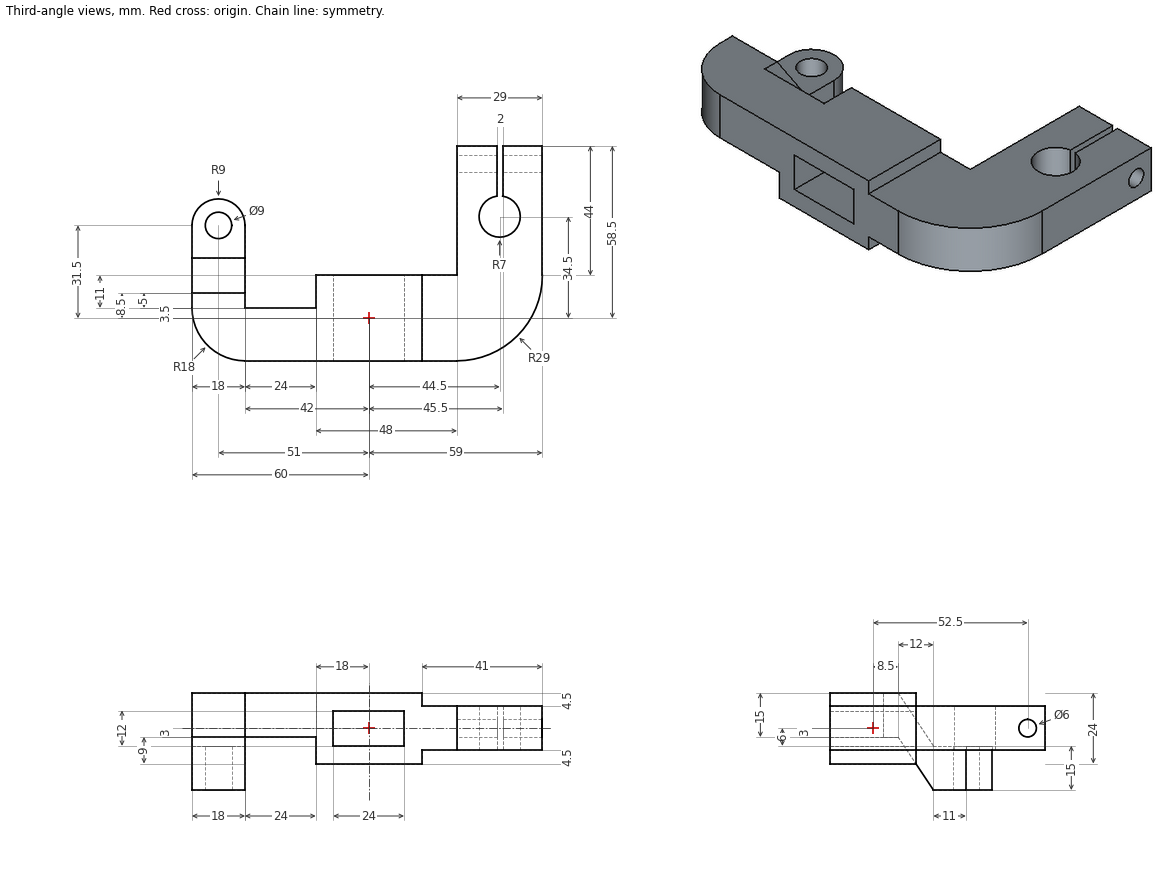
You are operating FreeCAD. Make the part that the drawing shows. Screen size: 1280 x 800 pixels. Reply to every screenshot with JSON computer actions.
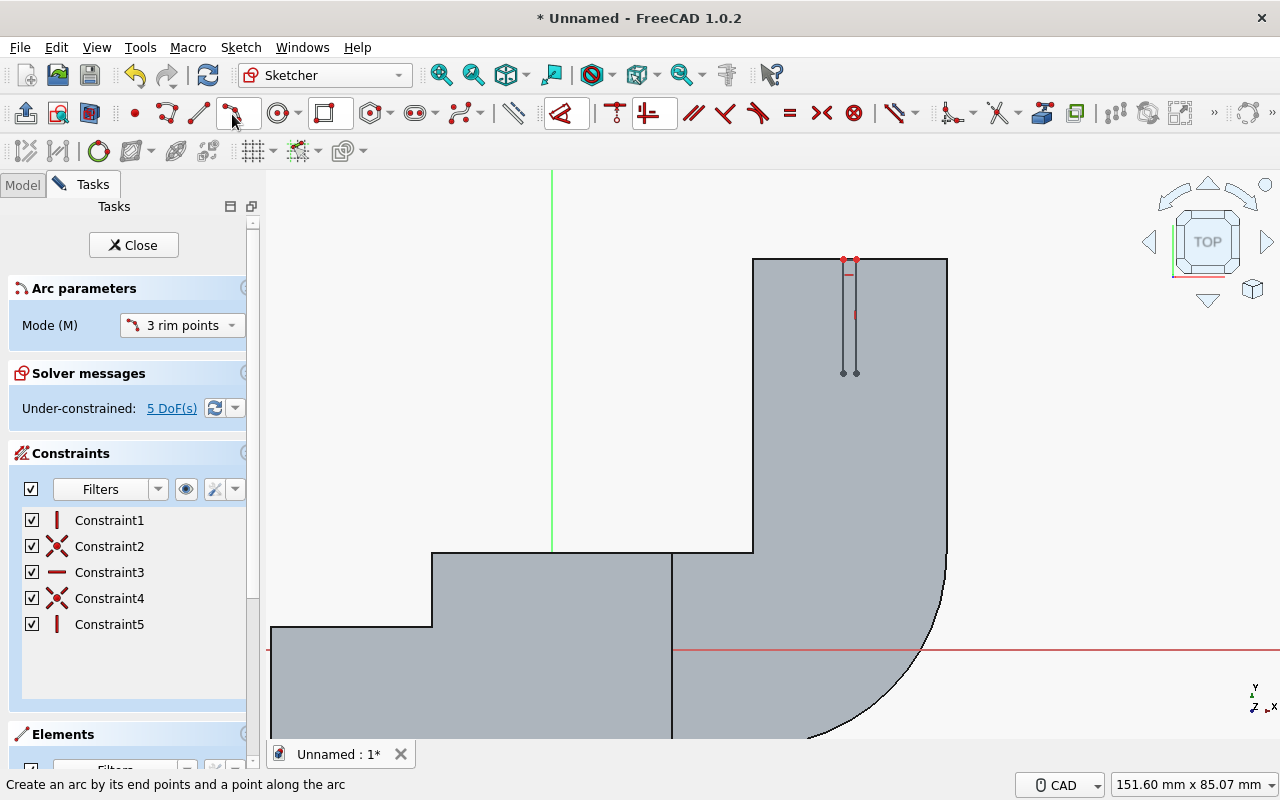
{"action": "left_click", "coordinate": [843, 374]}
{"action": "left_click", "coordinate": [856, 374]}
{"action": "left_click", "coordinate": [850, 466]}
{"action": "key", "text": "Escape"}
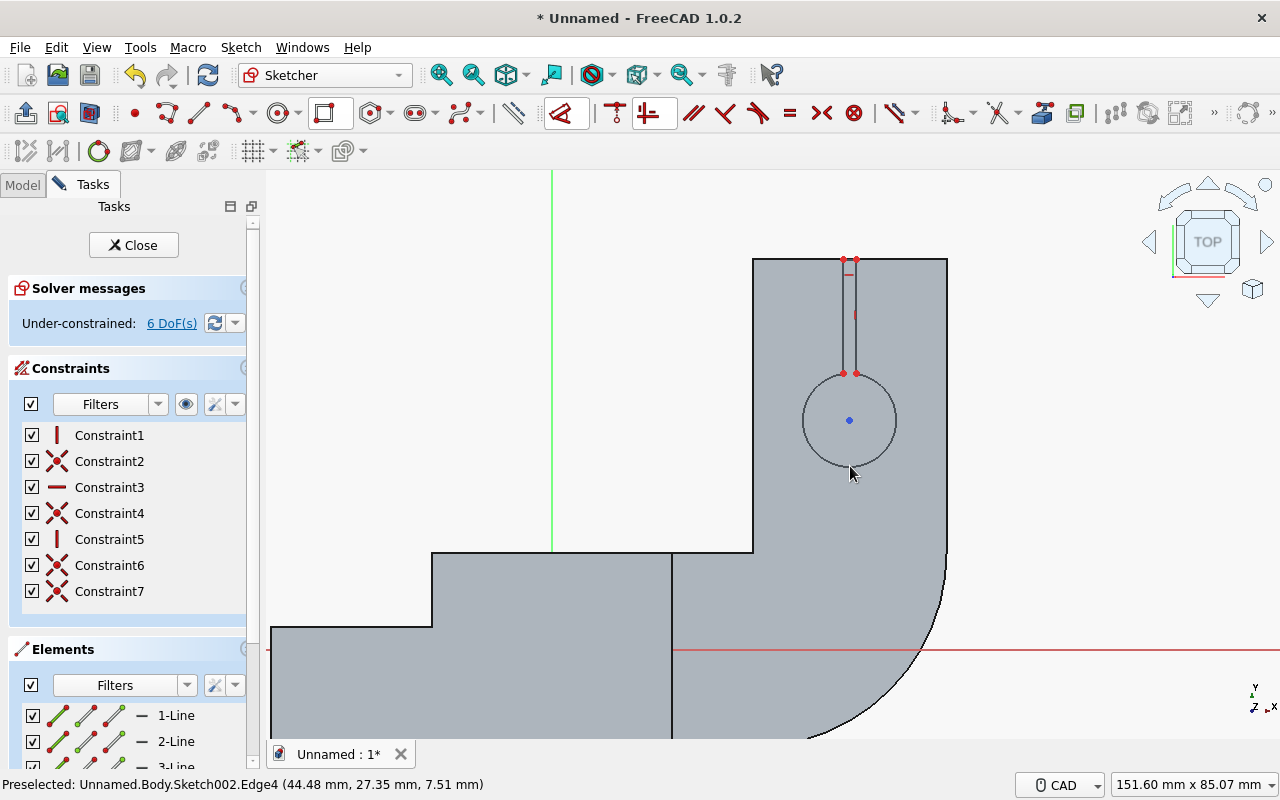
{"action": "left_click", "coordinate": [806, 437]}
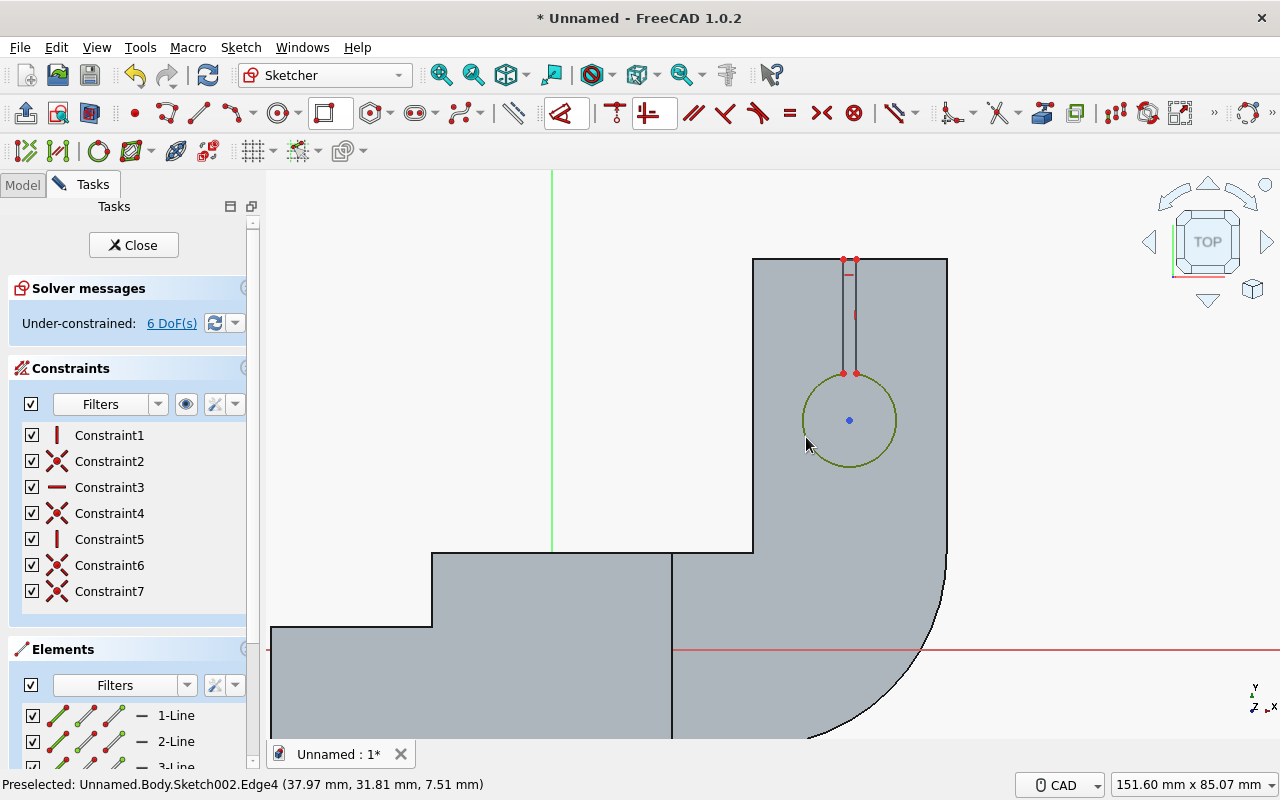
{"action": "key", "text": "k r"}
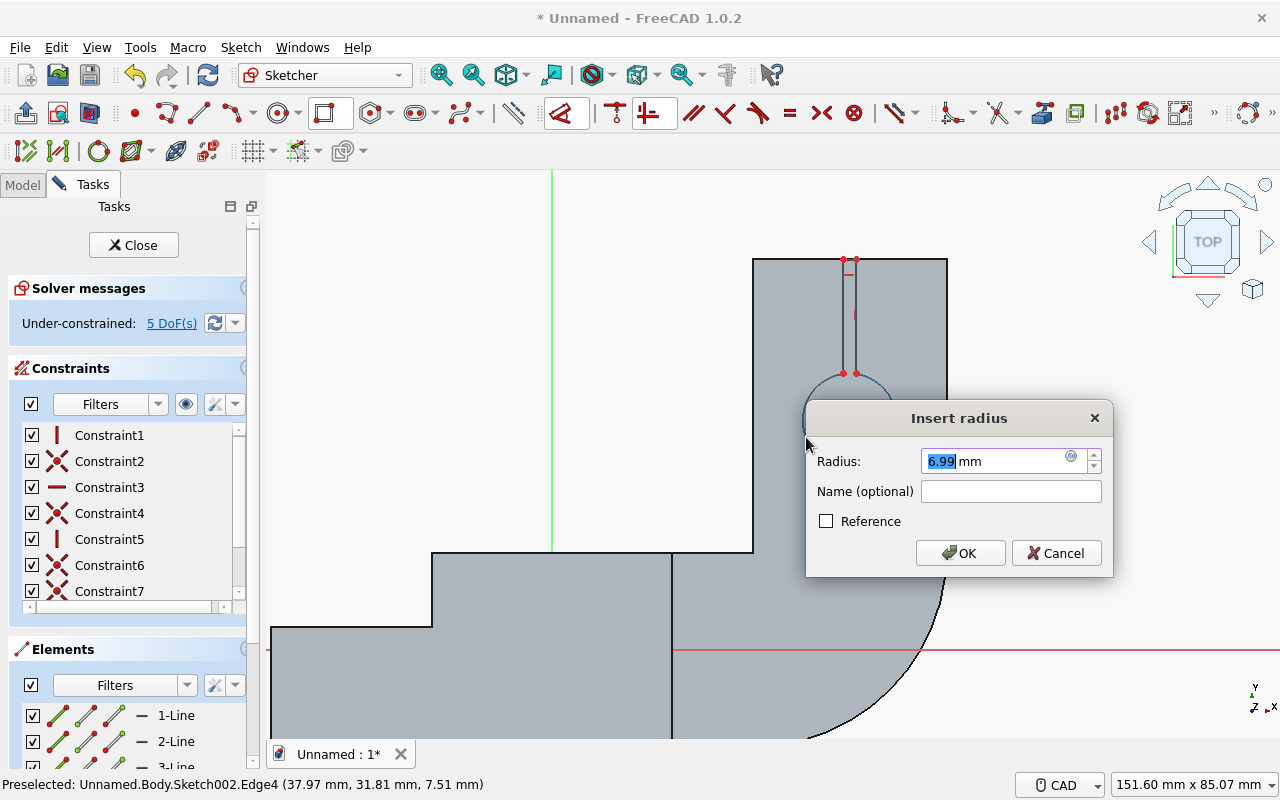
{"action": "type", "text": "7"}
{"action": "key", "text": "Return"}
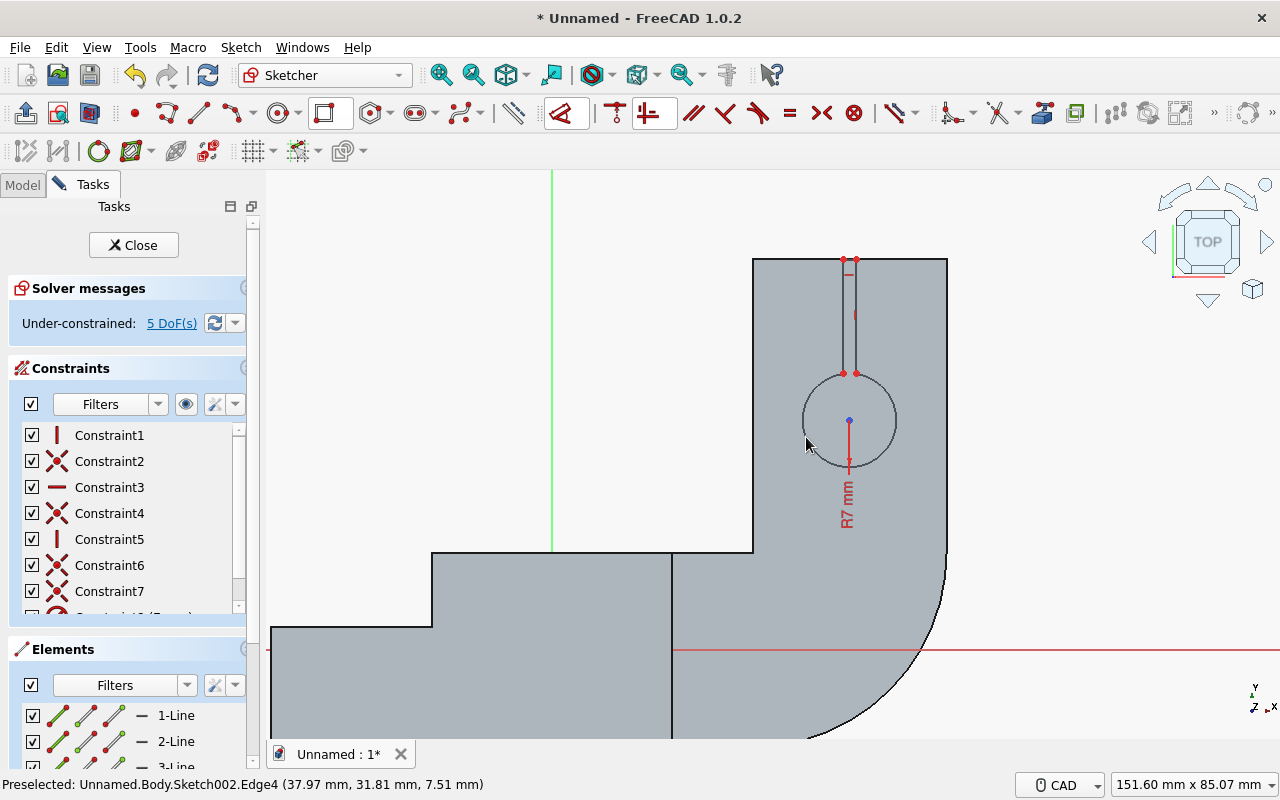
{"action": "scroll", "coordinate": [849, 260], "scroll_direction": "up", "scroll_amount": 6}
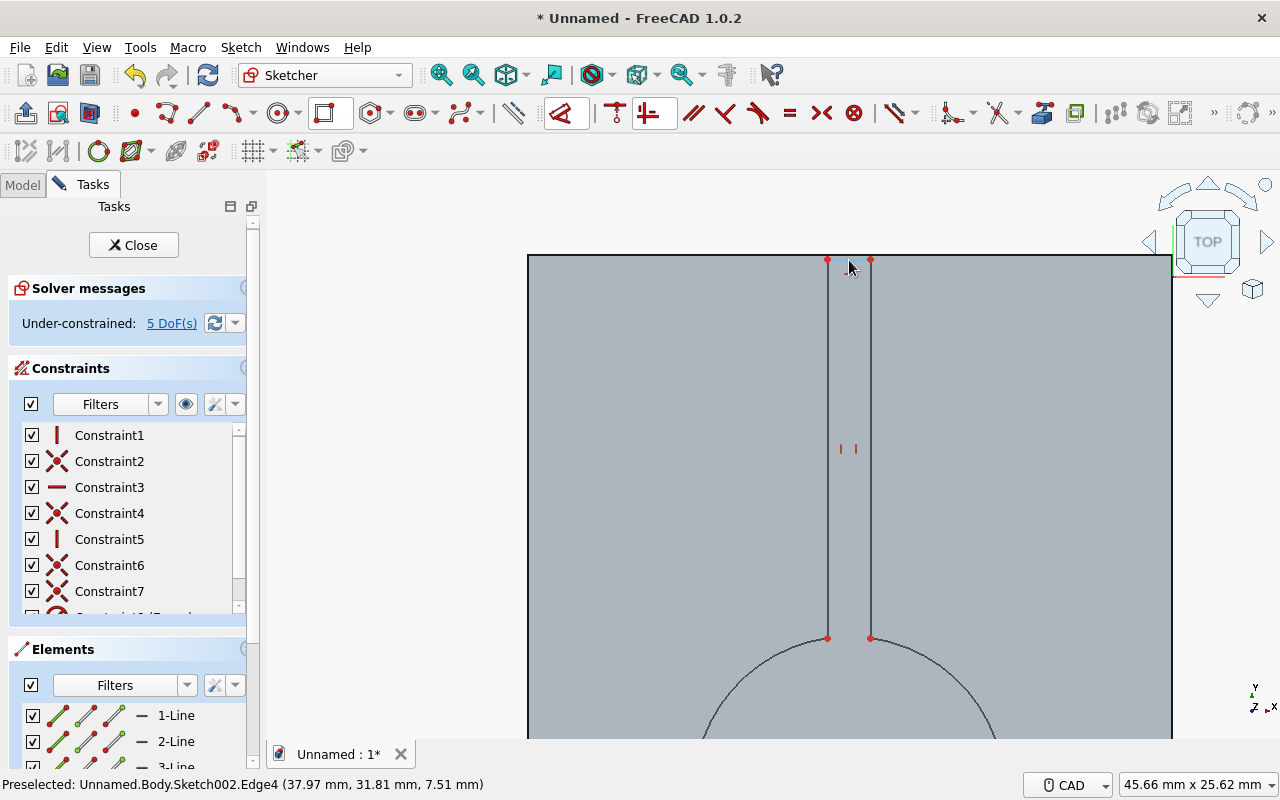
{"action": "left_click", "coordinate": [849, 260]}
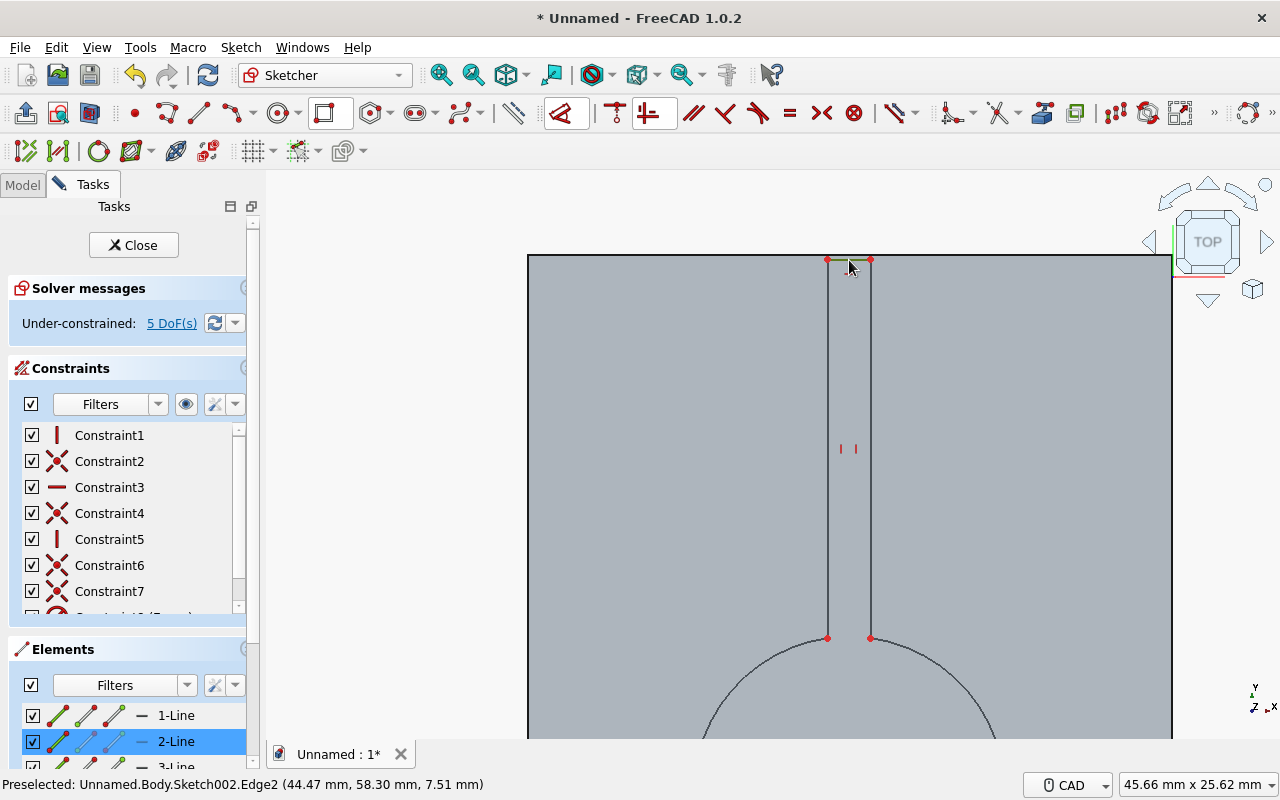
{"action": "key", "text": "l"}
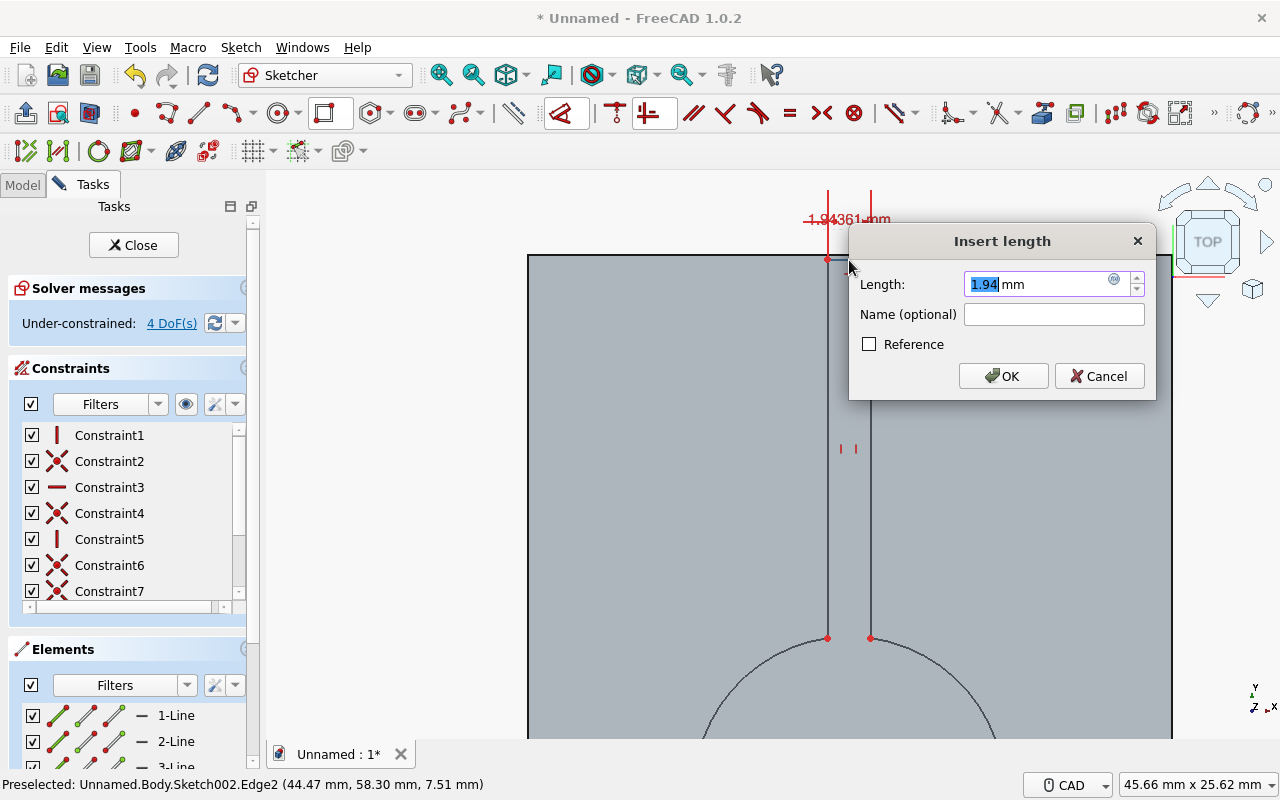
{"action": "type", "text": "2"}
{"action": "key", "text": "Return"}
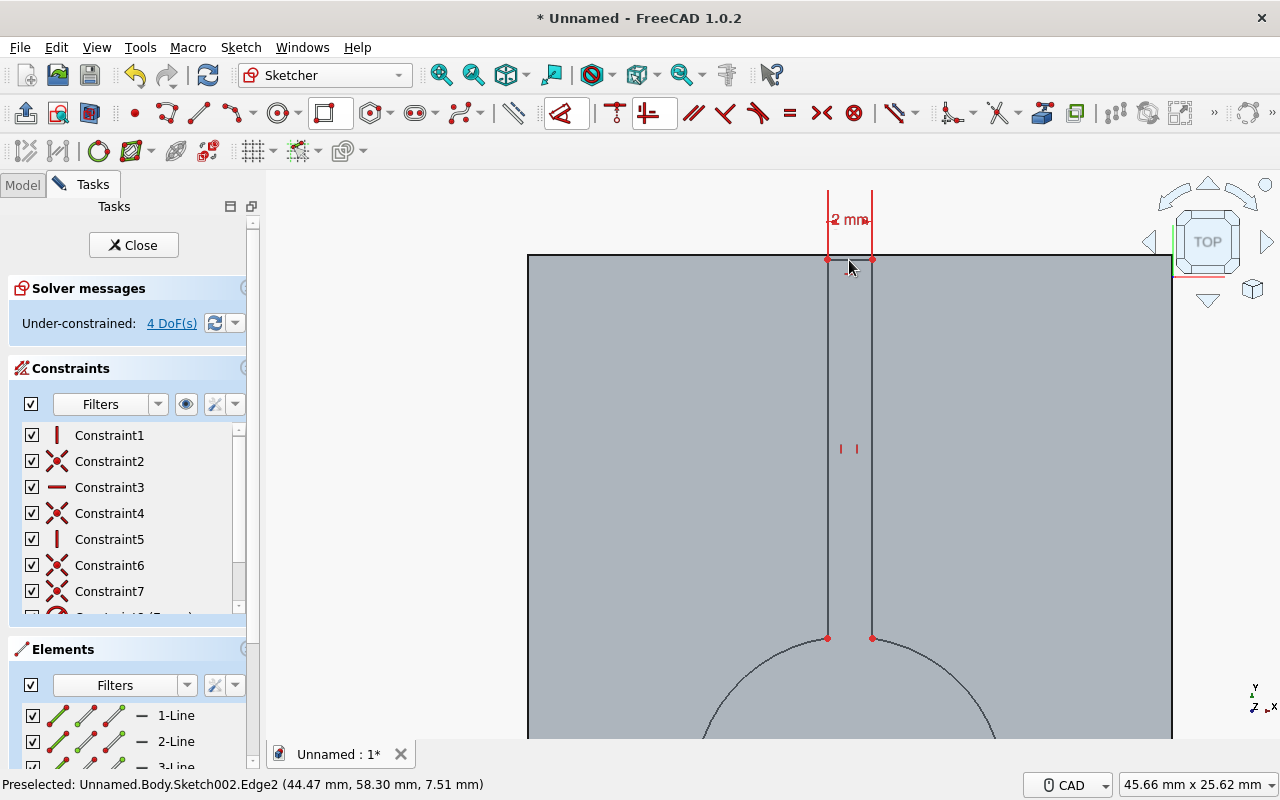
{"action": "left_click", "coordinate": [872, 638]}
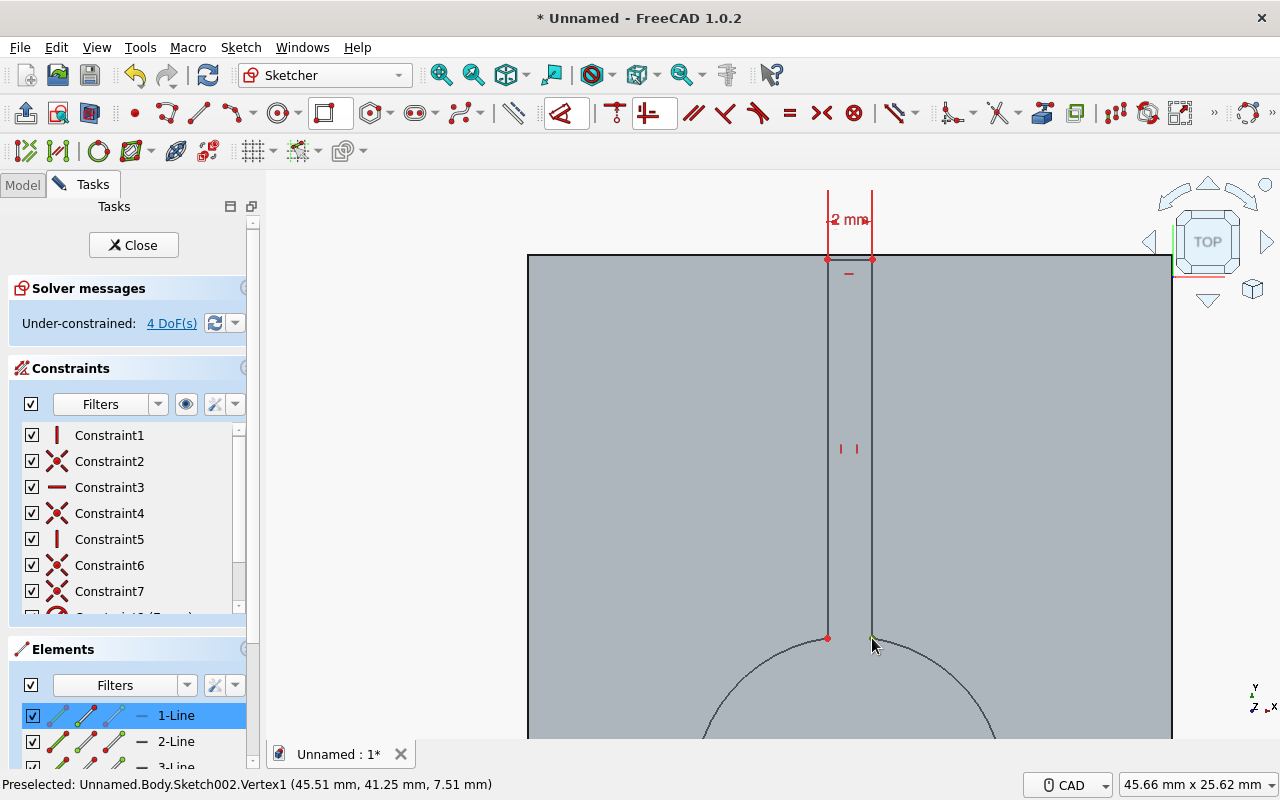
{"action": "key", "text": "l"}